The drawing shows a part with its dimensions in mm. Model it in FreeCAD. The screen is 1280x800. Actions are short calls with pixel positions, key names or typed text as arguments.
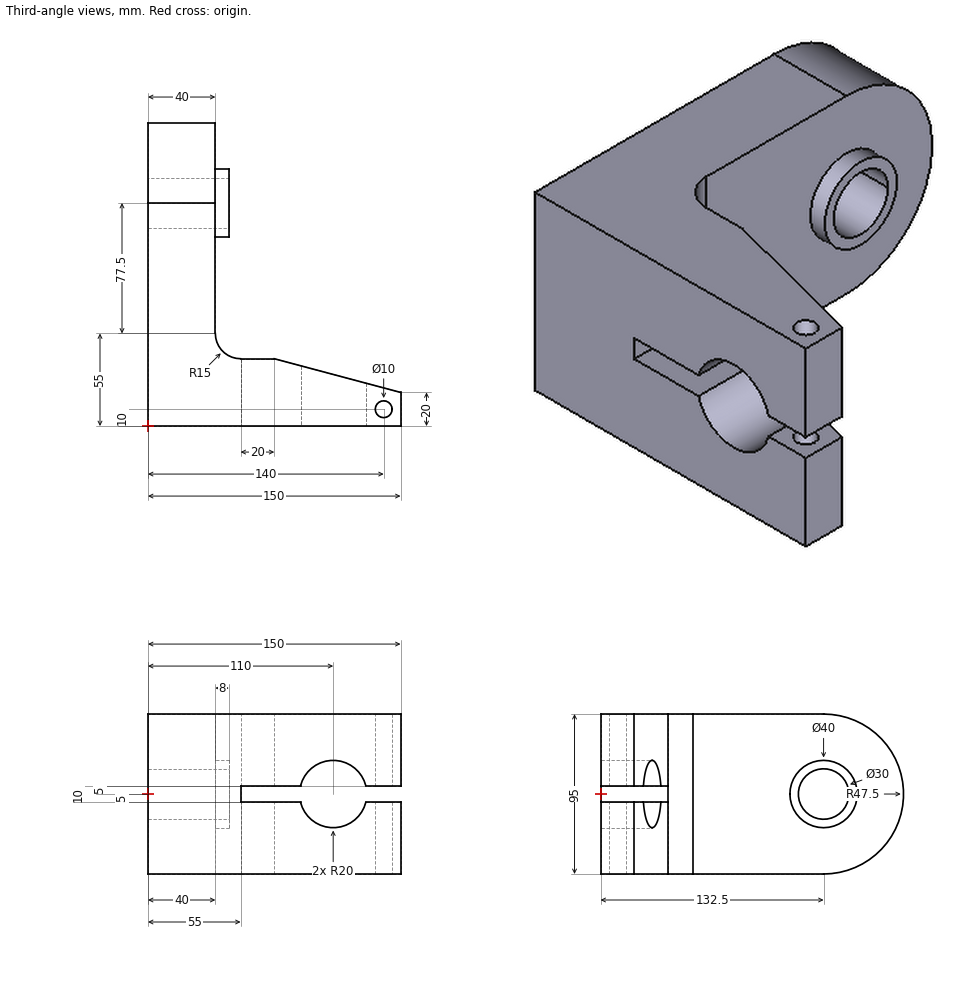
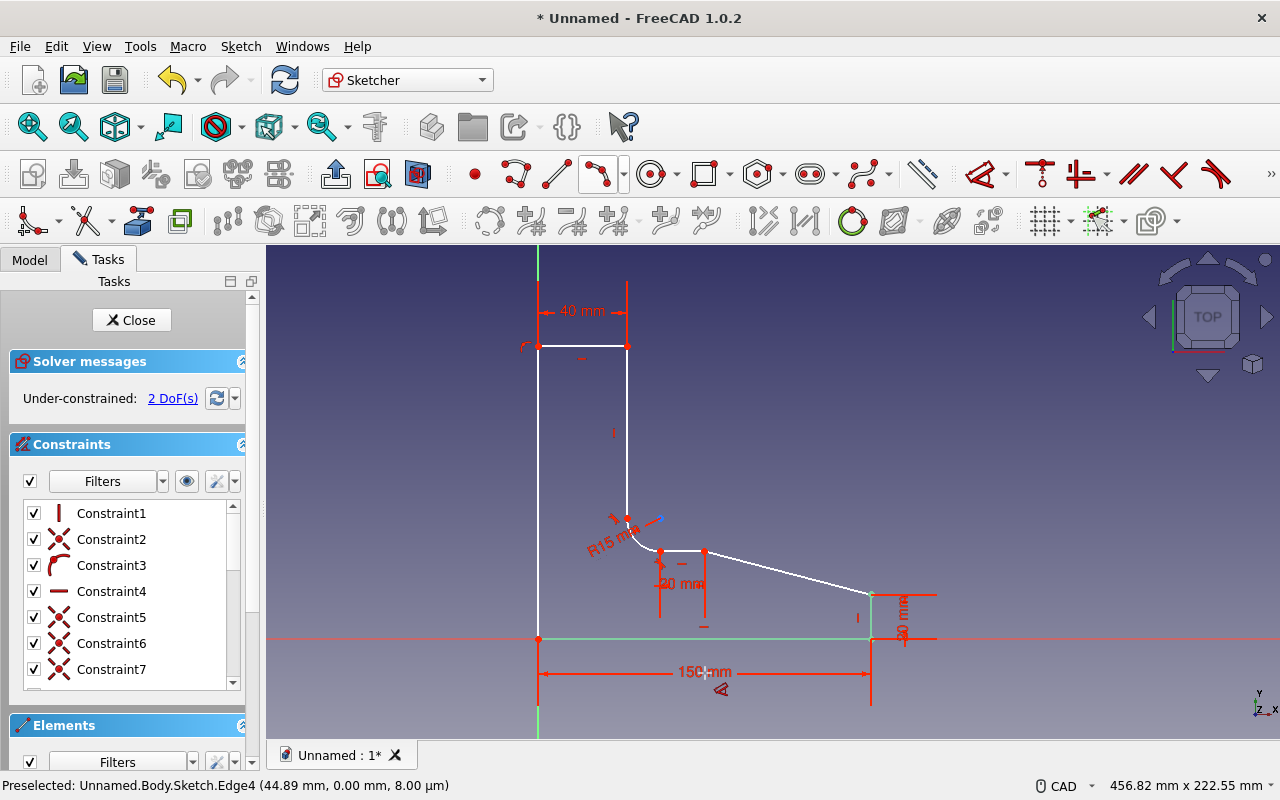
click(627, 518)
click(504, 579)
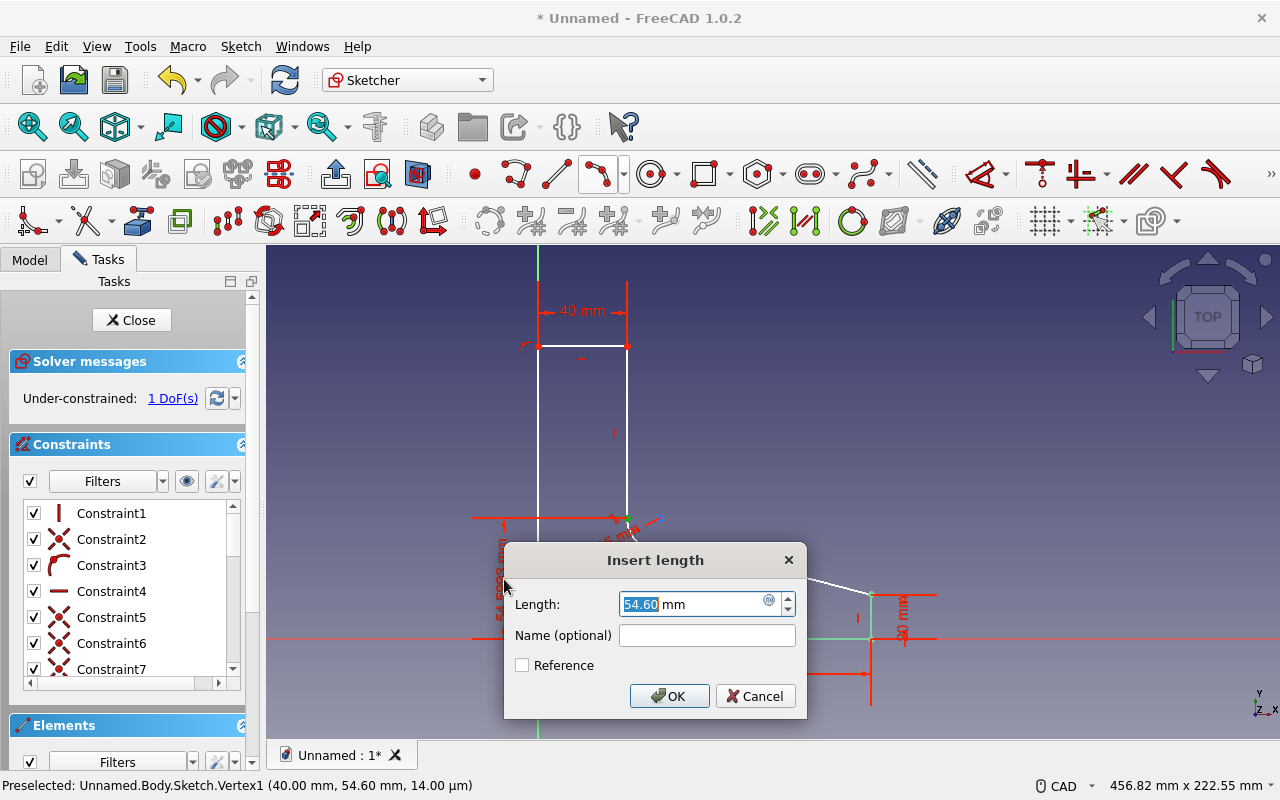
text(55)
key(Return)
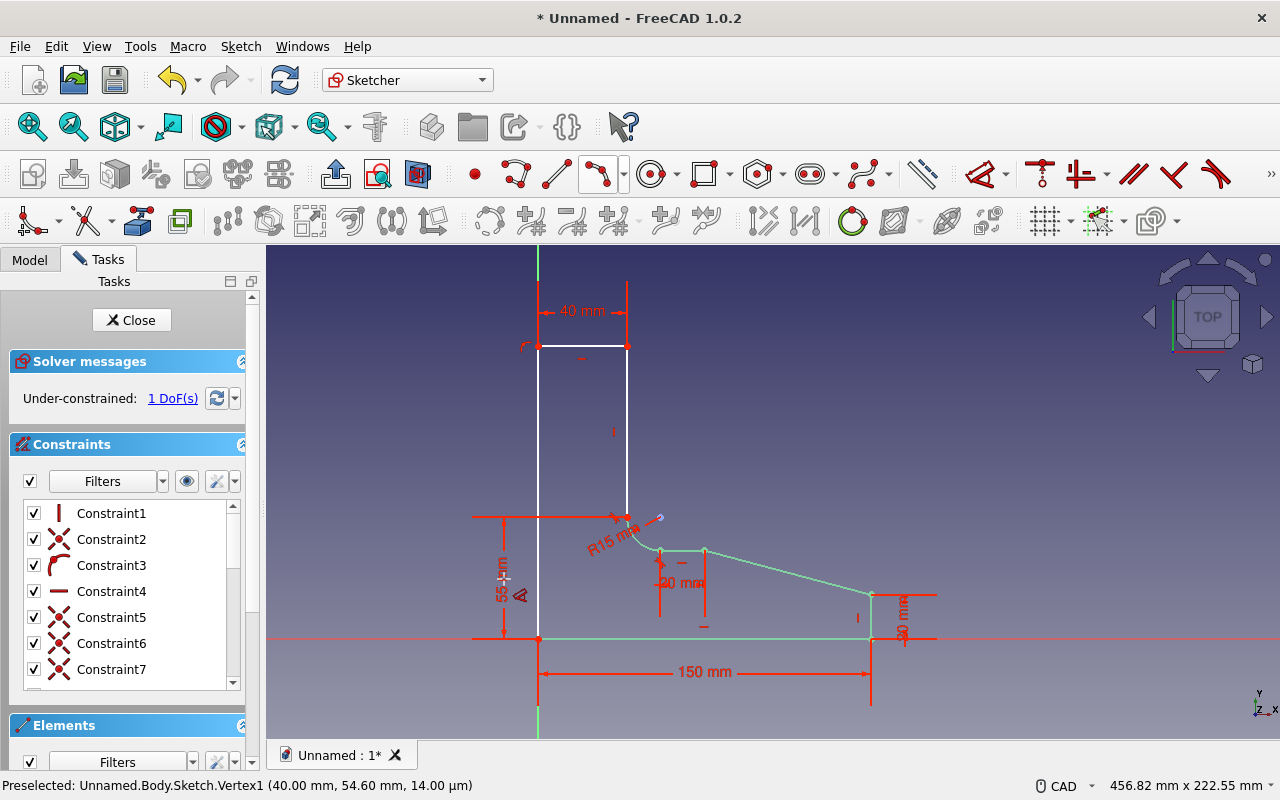
click(627, 466)
click(593, 432)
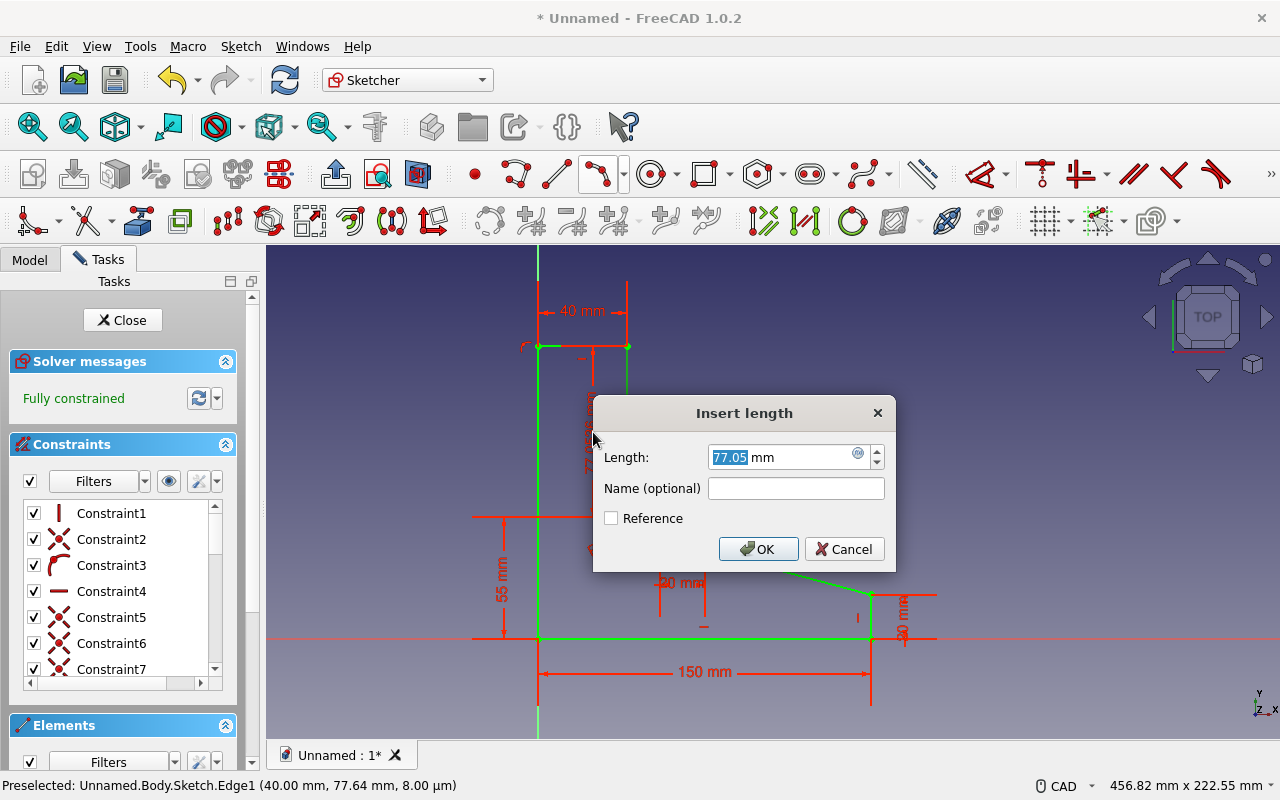
text(77.5)
key(Return)
key(Escape)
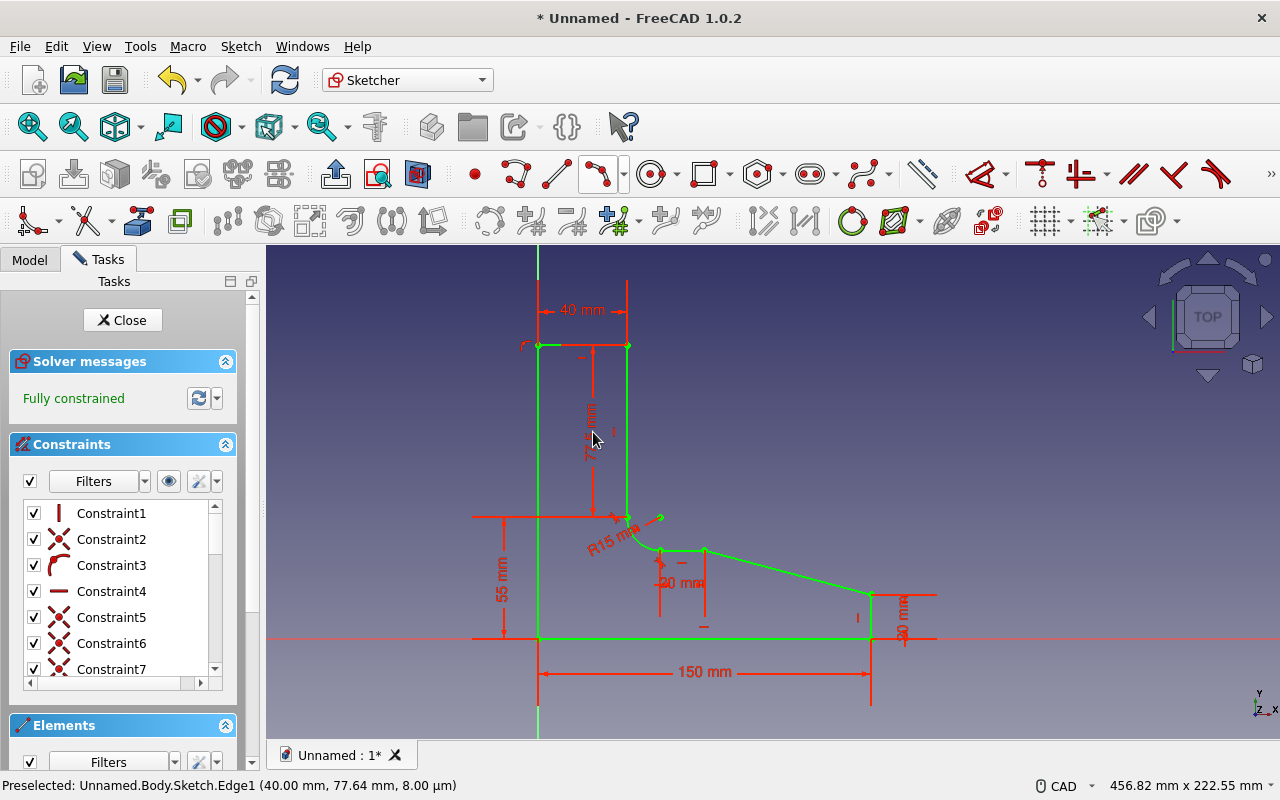
click(123, 320)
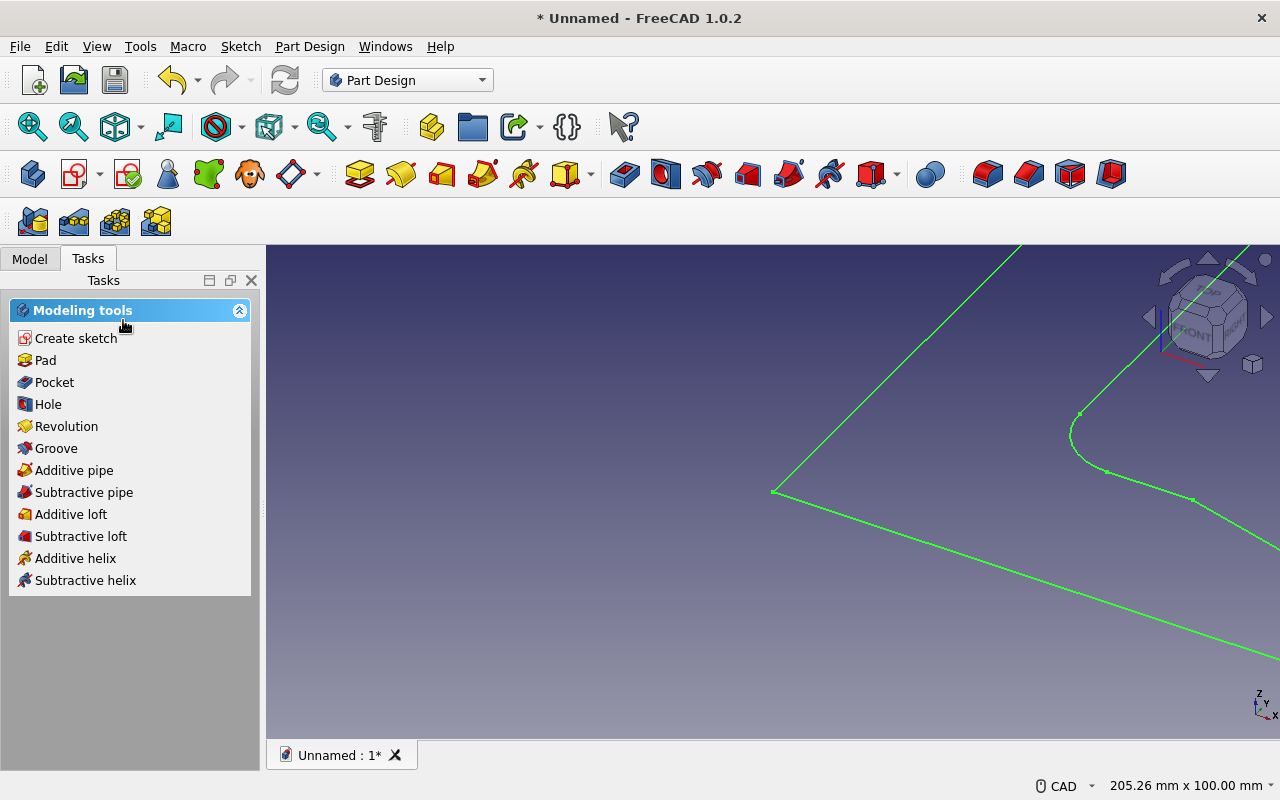
click(360, 174)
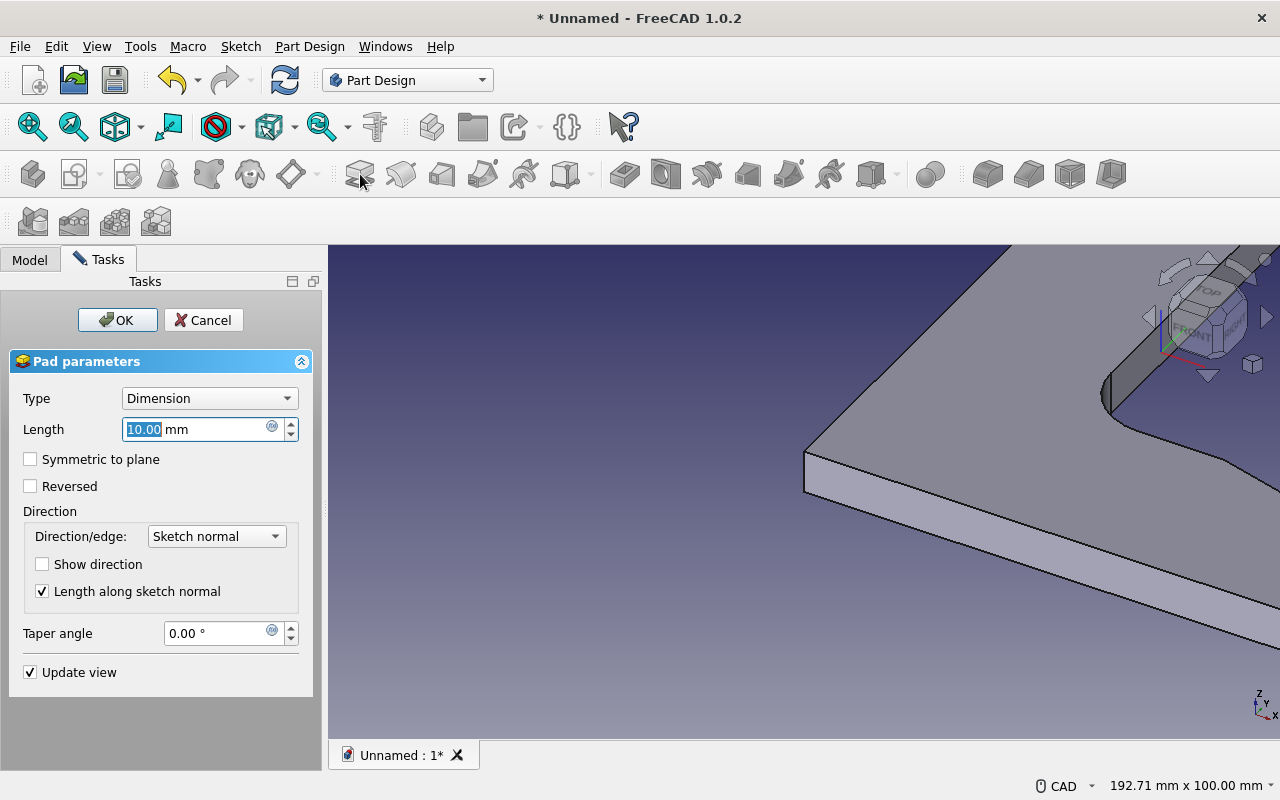
text(95)
key(Tab)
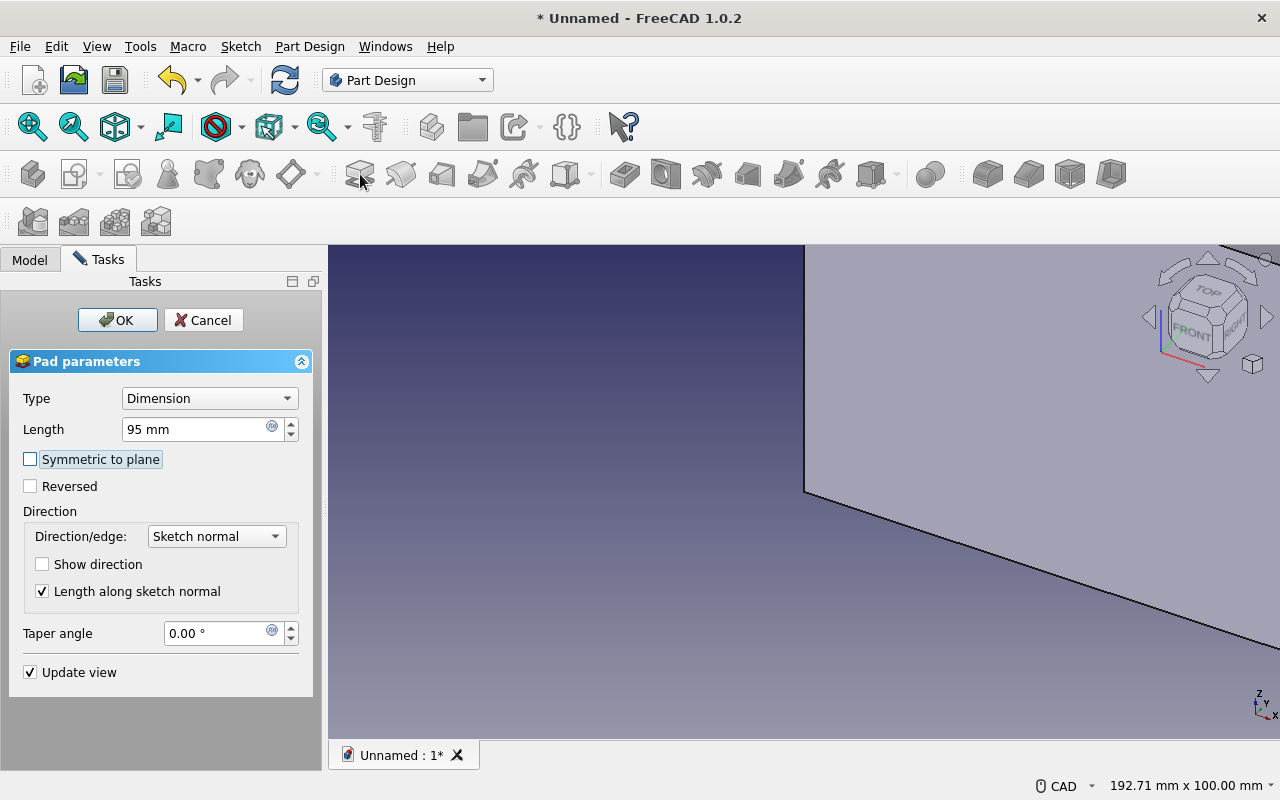
click(31, 459)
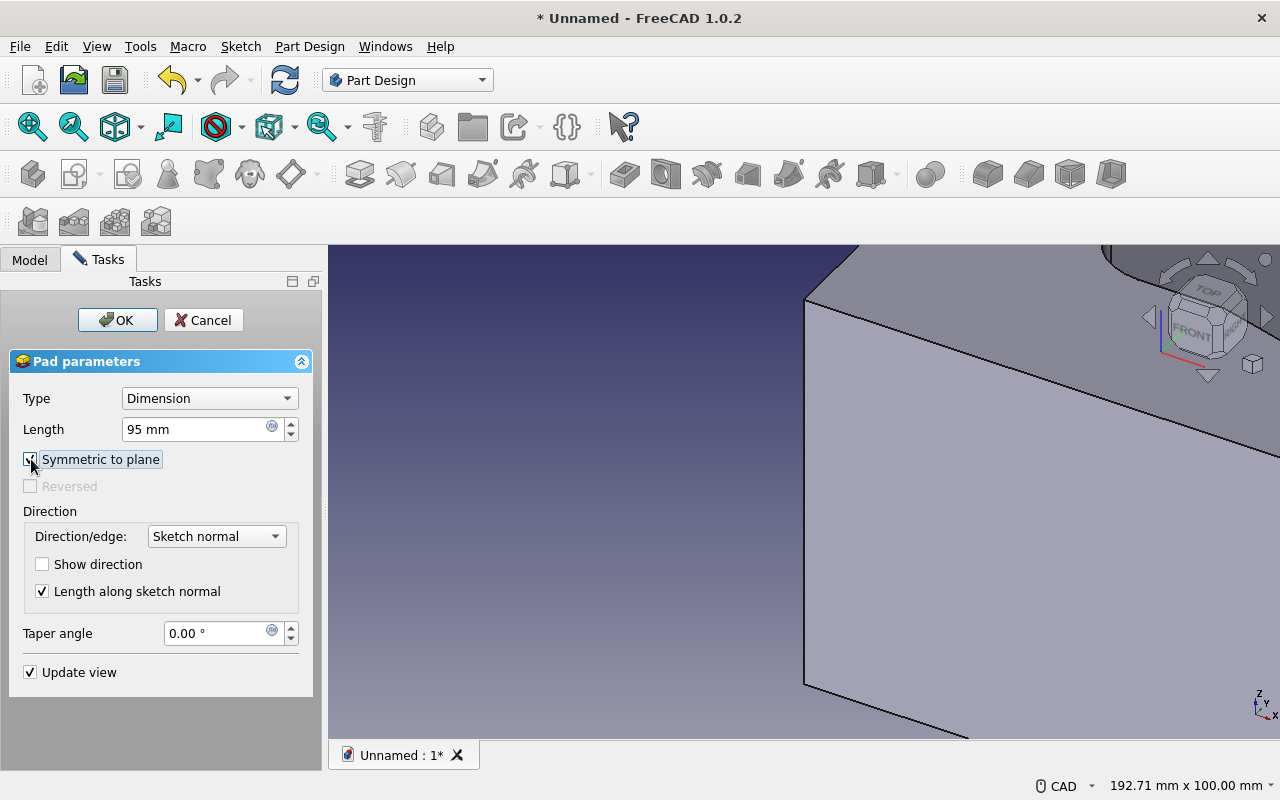
click(118, 320)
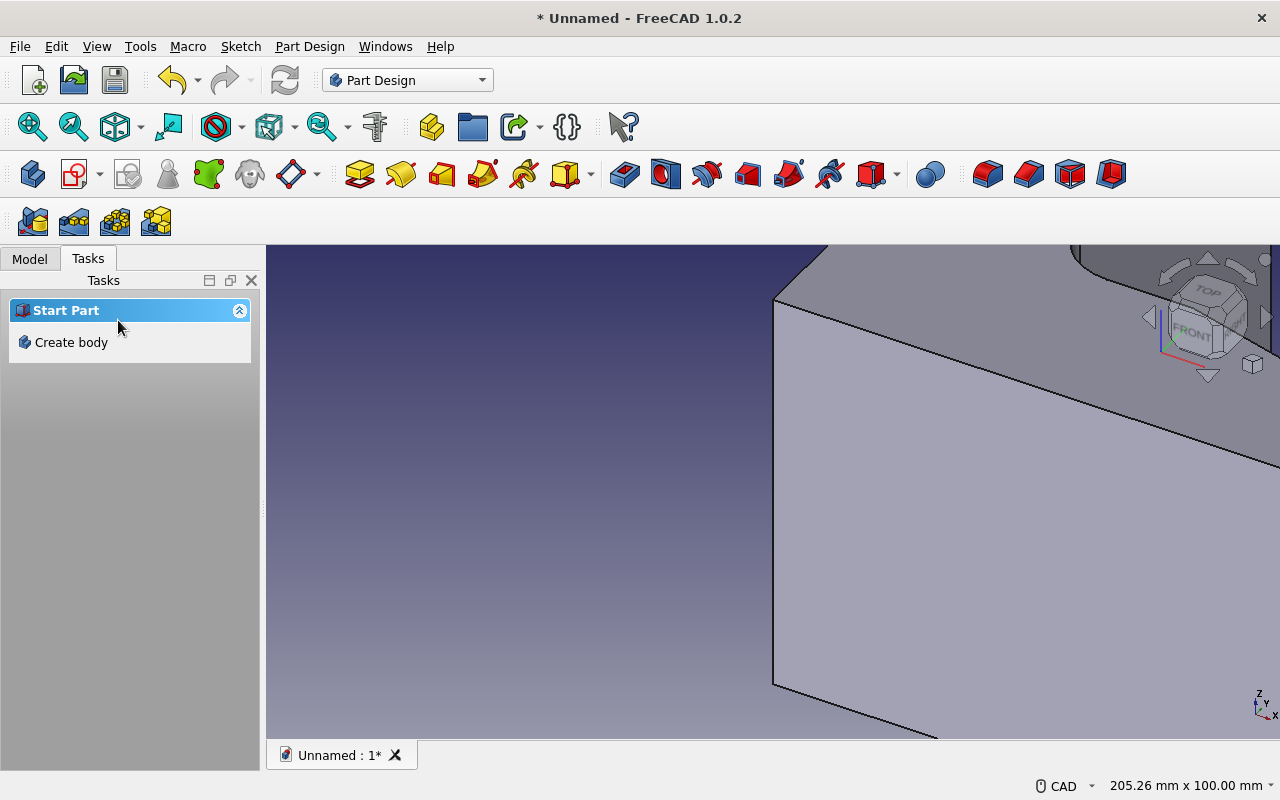
click(33, 128)